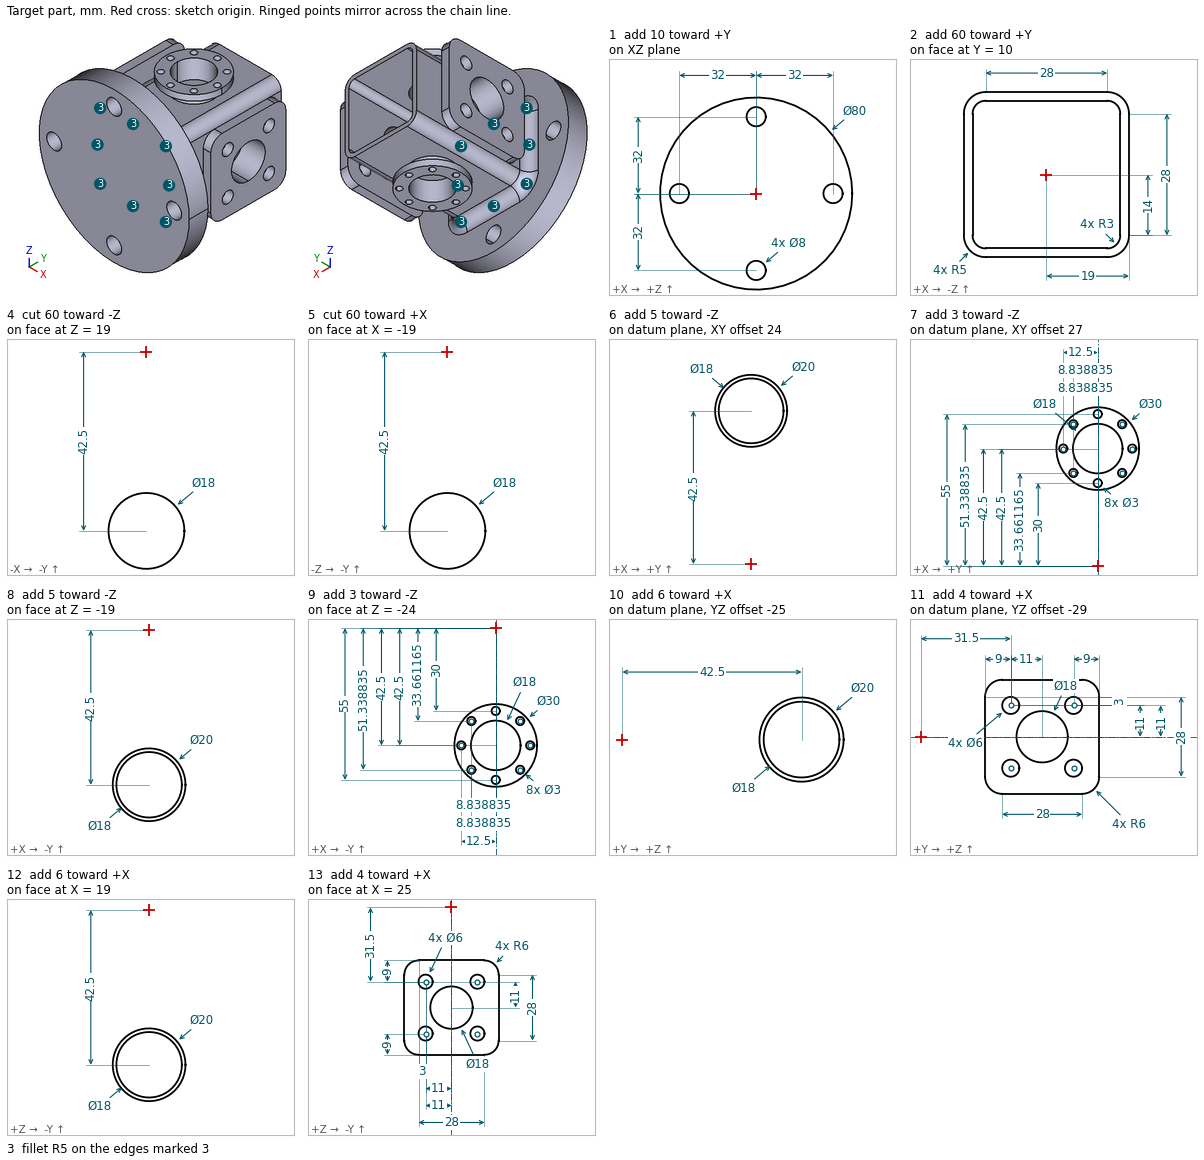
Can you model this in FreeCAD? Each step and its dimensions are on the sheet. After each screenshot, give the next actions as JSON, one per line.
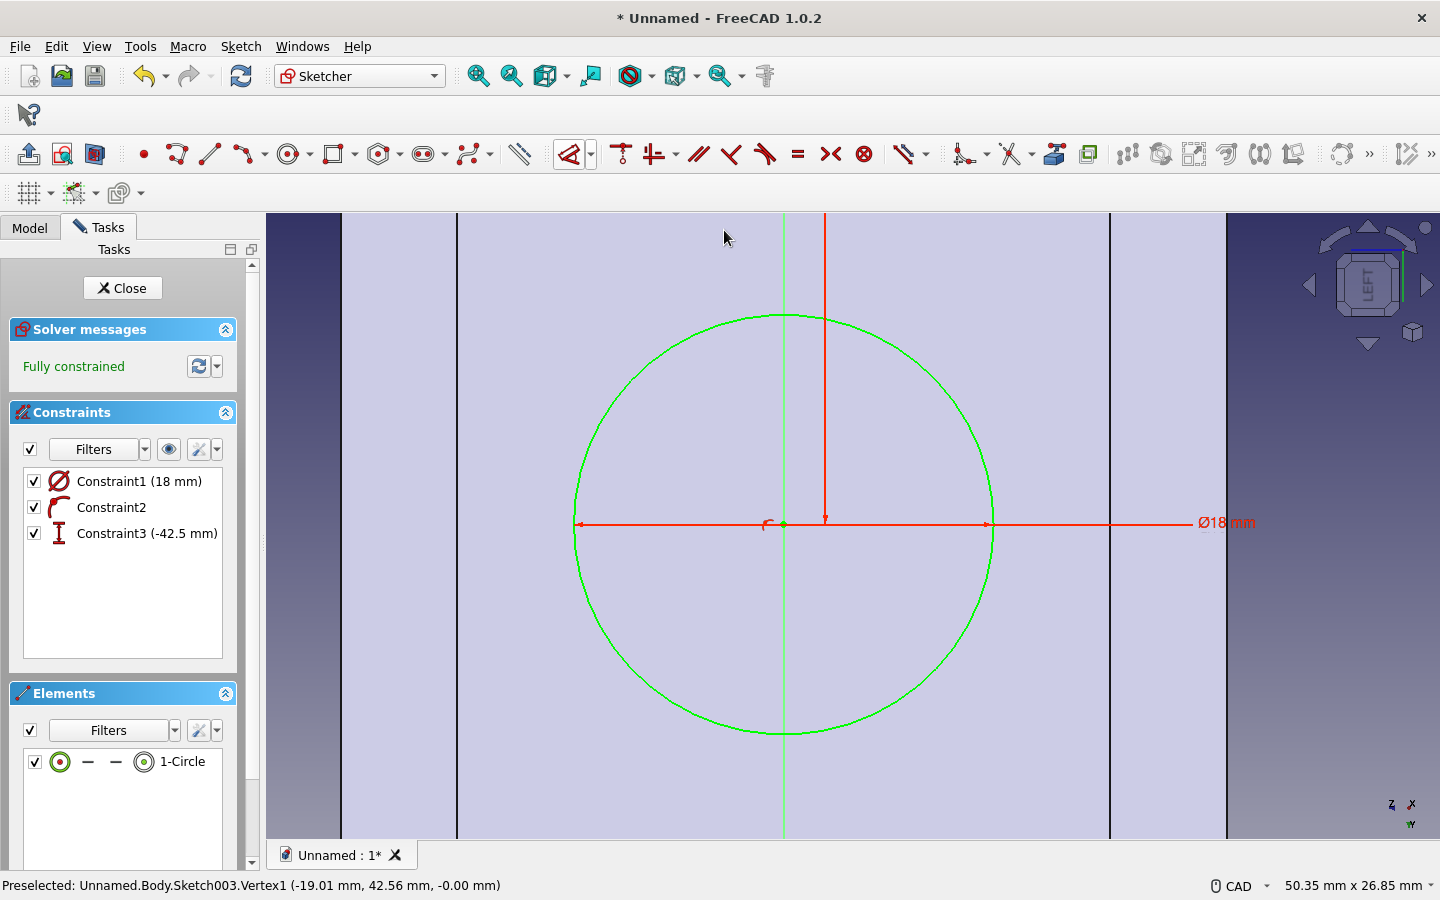
{"action": "left_click", "coordinate": [123, 288]}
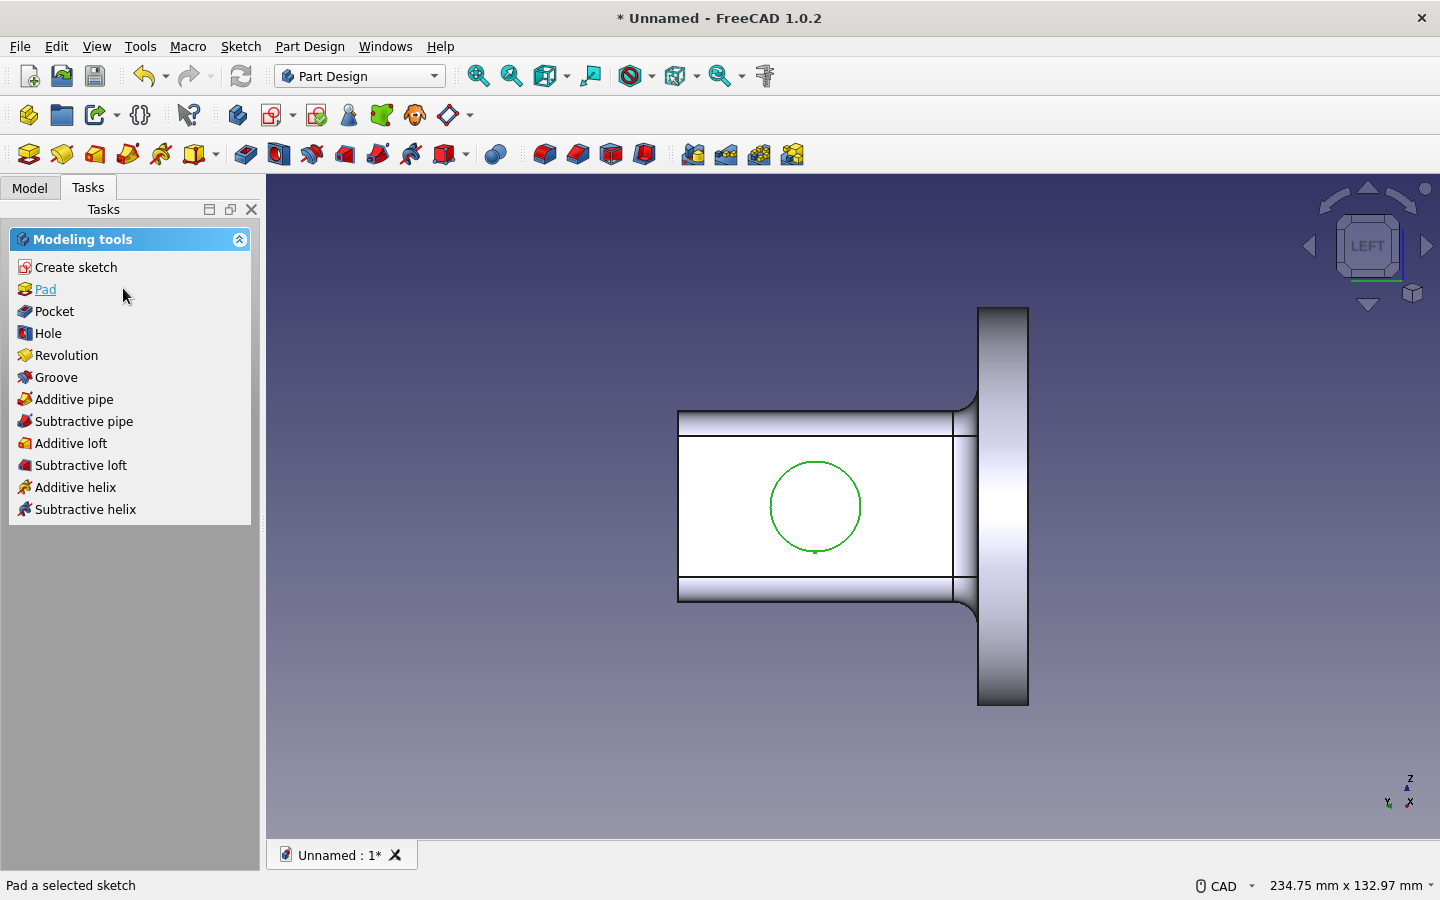
{"action": "left_click", "coordinate": [246, 154]}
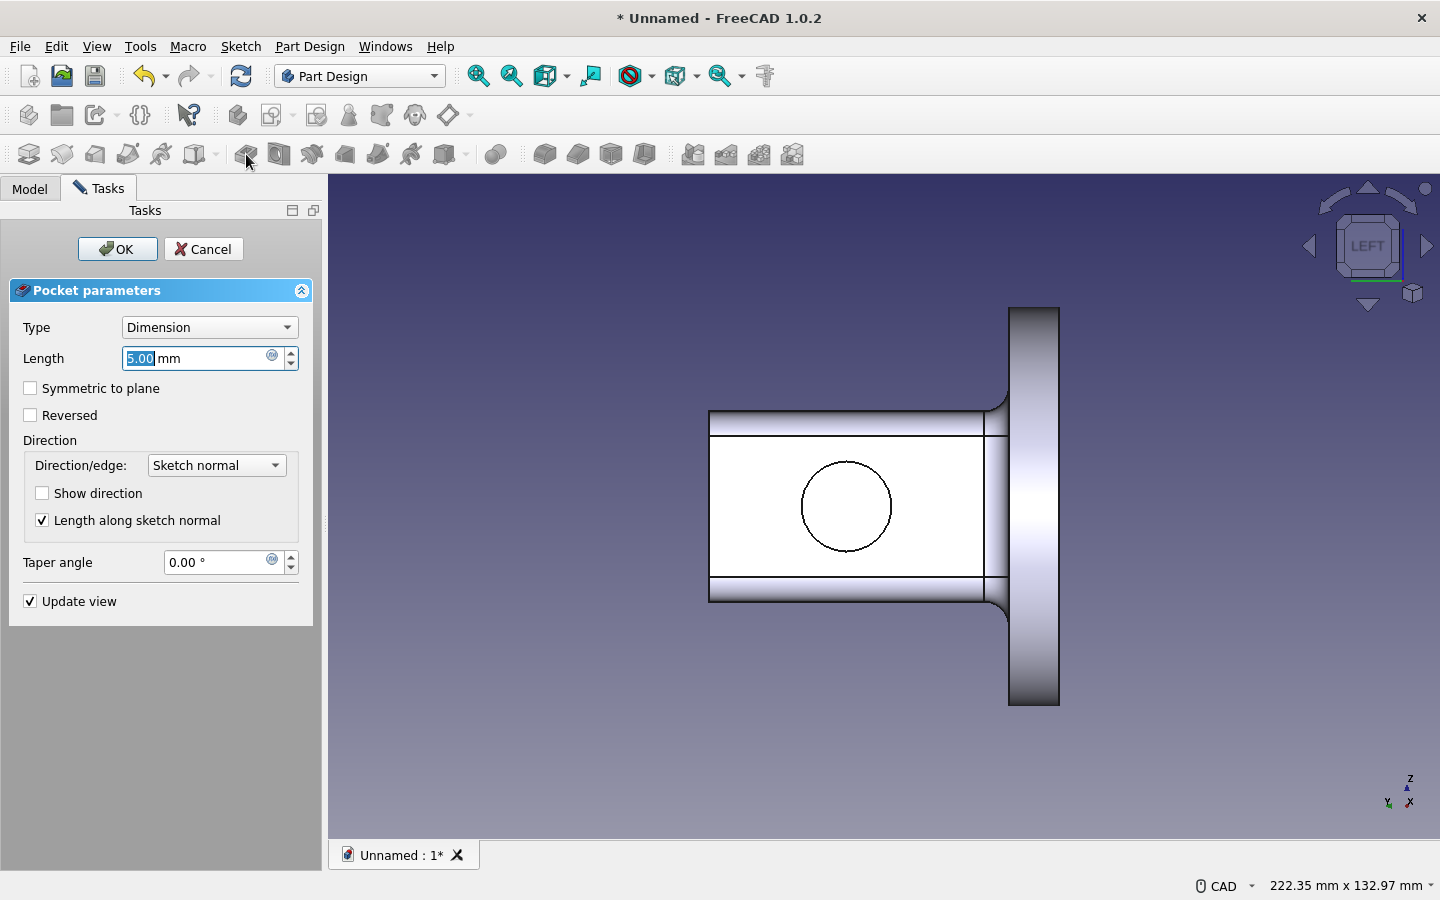
{"action": "type", "text": "60"}
{"action": "key", "text": "Tab"}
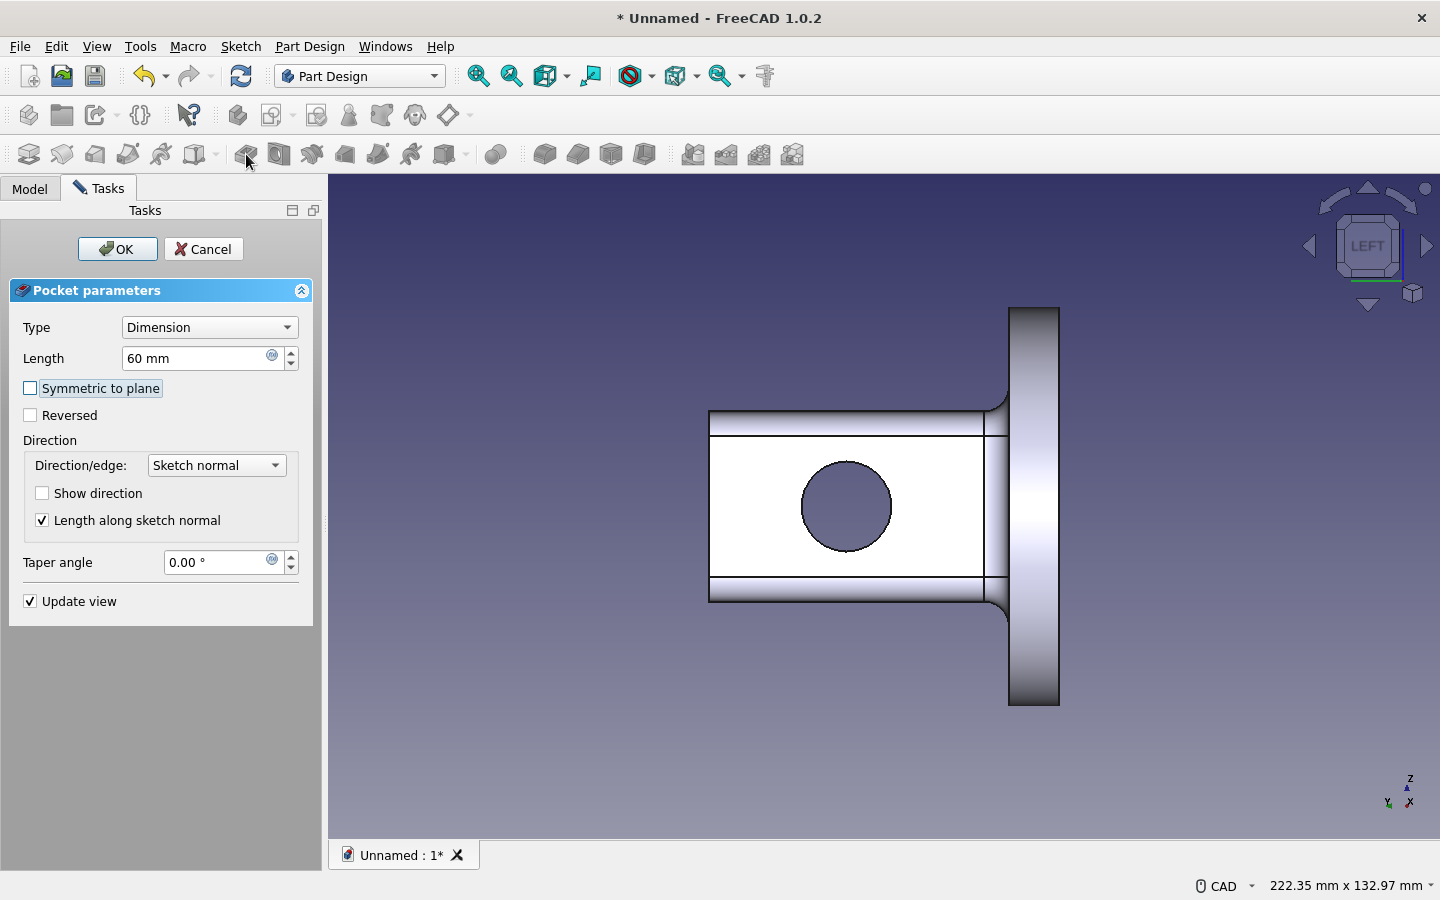
{"action": "left_click", "coordinate": [118, 249]}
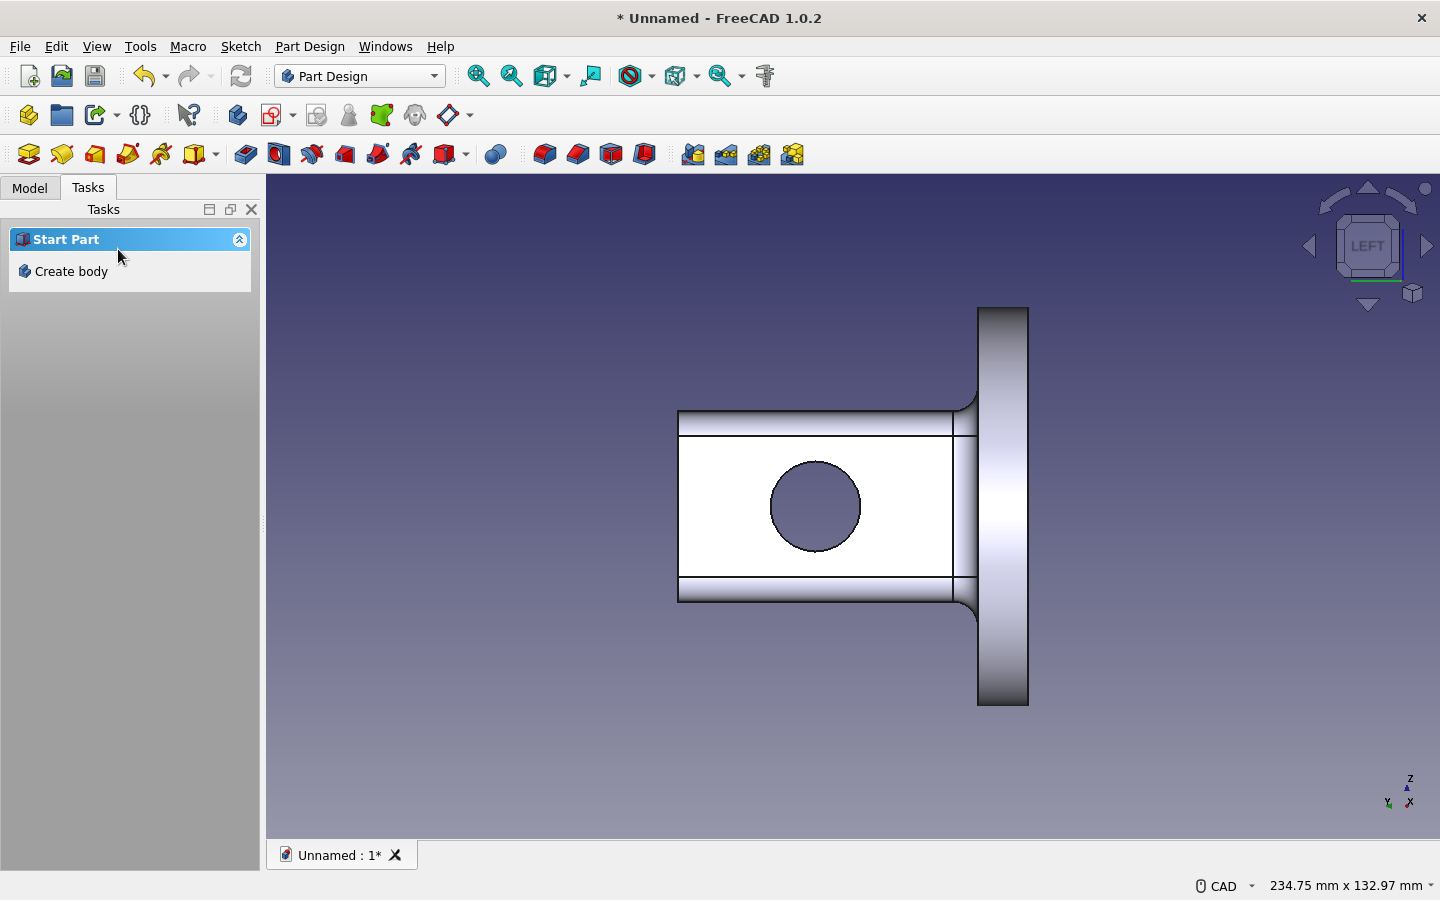
{"action": "left_click", "coordinate": [30, 188]}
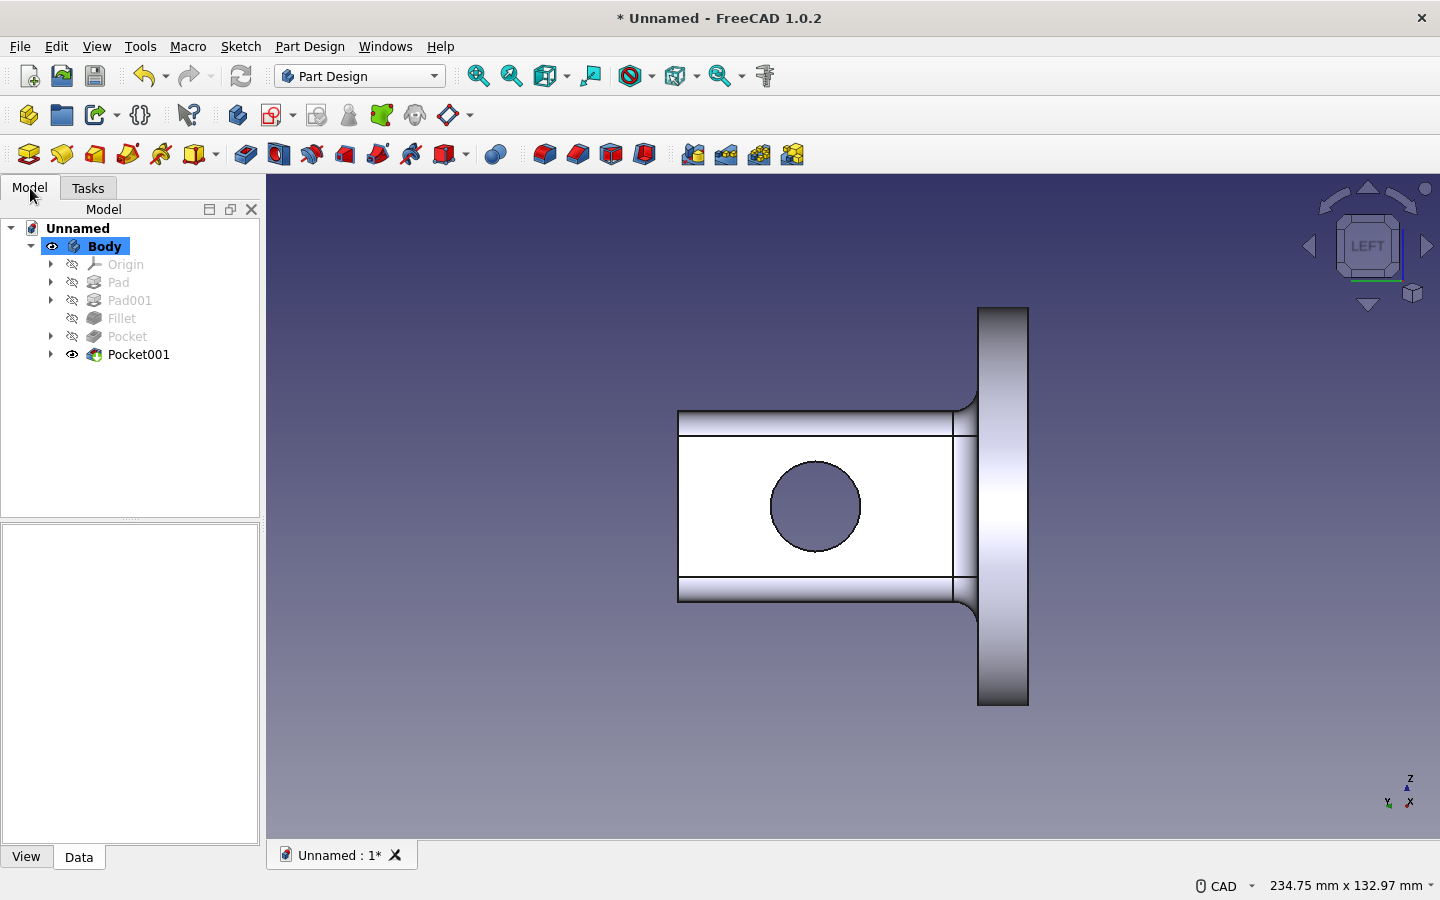
{"action": "left_click", "coordinate": [51, 264]}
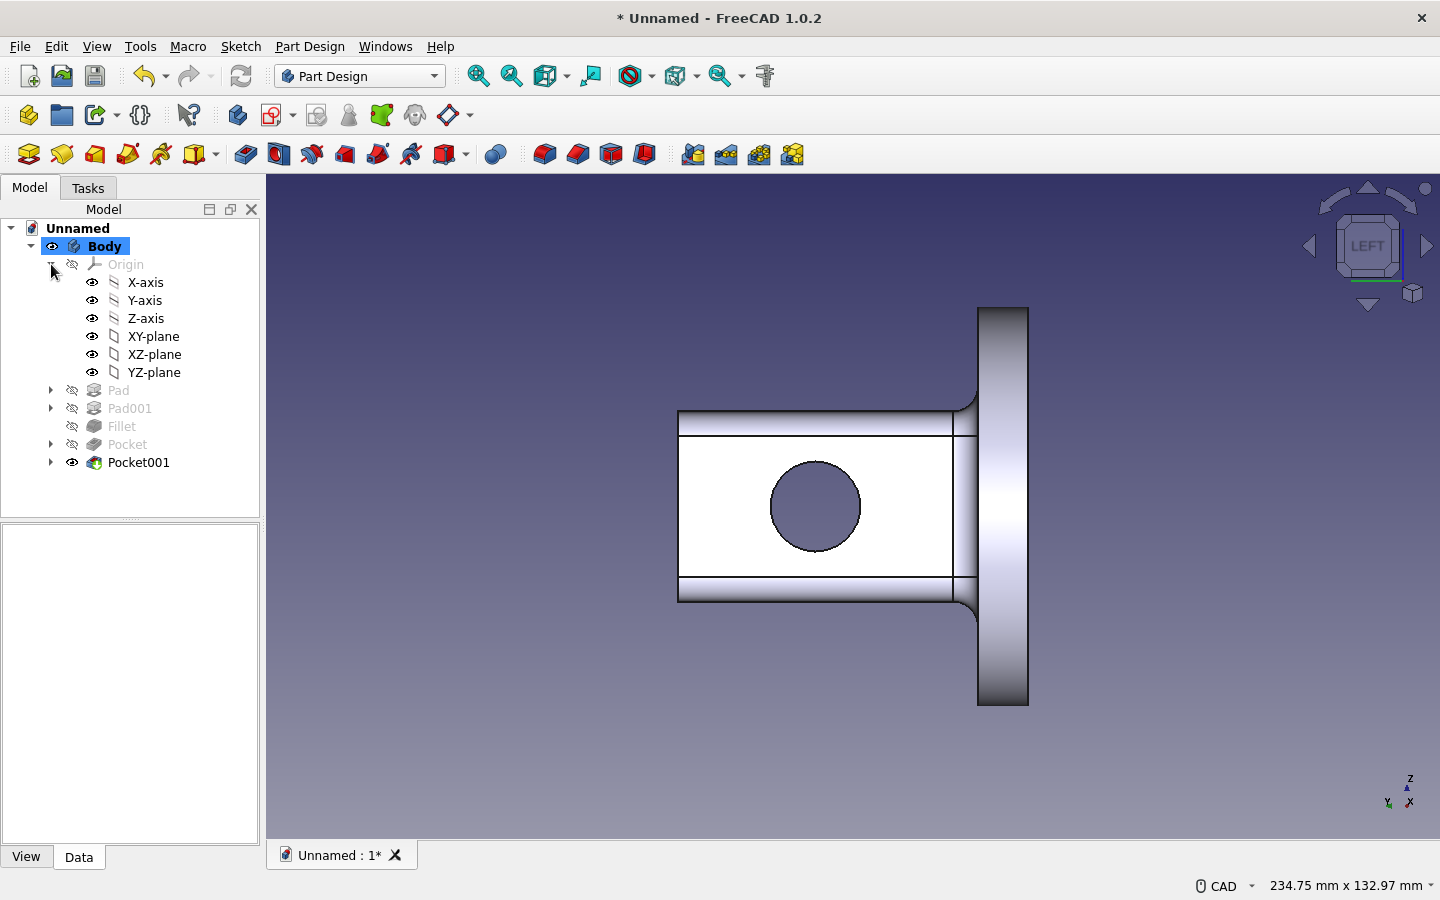
{"action": "left_click", "coordinate": [137, 336]}